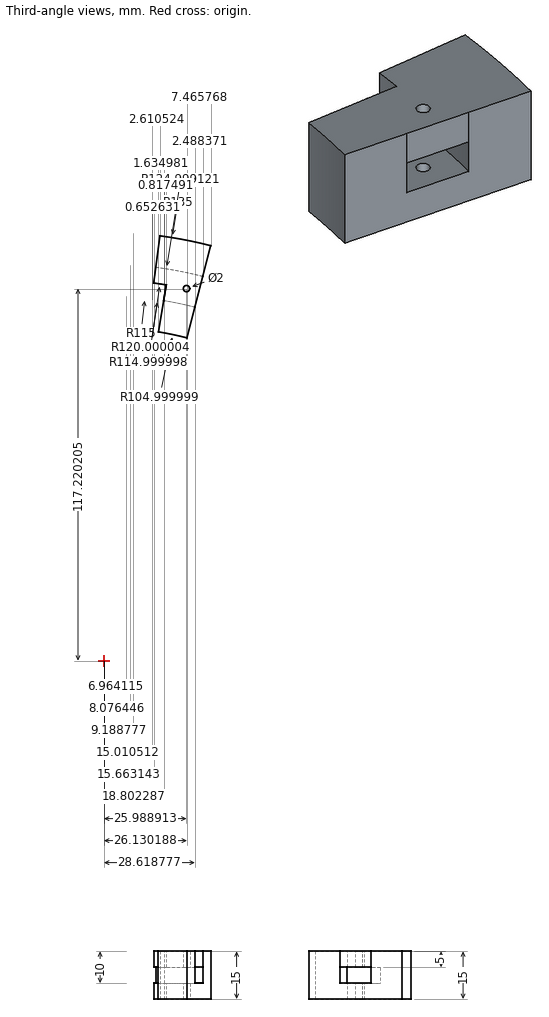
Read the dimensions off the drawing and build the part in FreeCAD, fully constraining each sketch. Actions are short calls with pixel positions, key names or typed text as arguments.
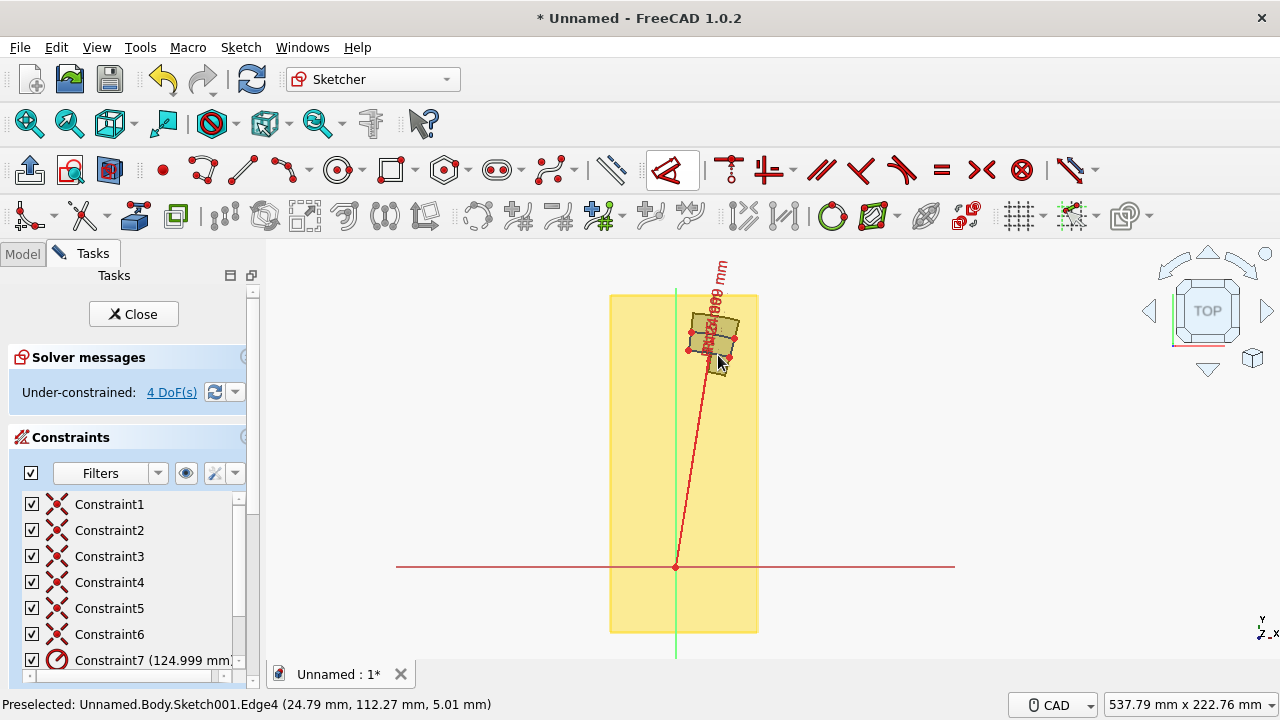
scroll(691, 332, up, 5)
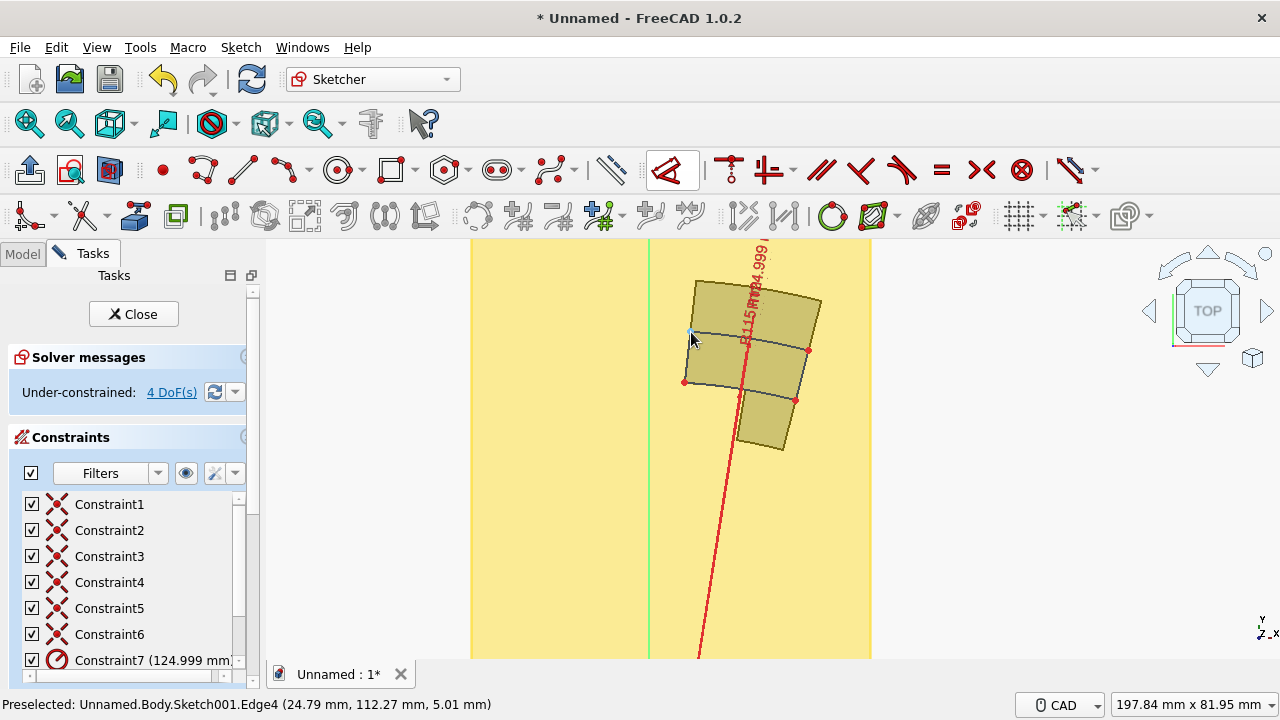
click(690, 332)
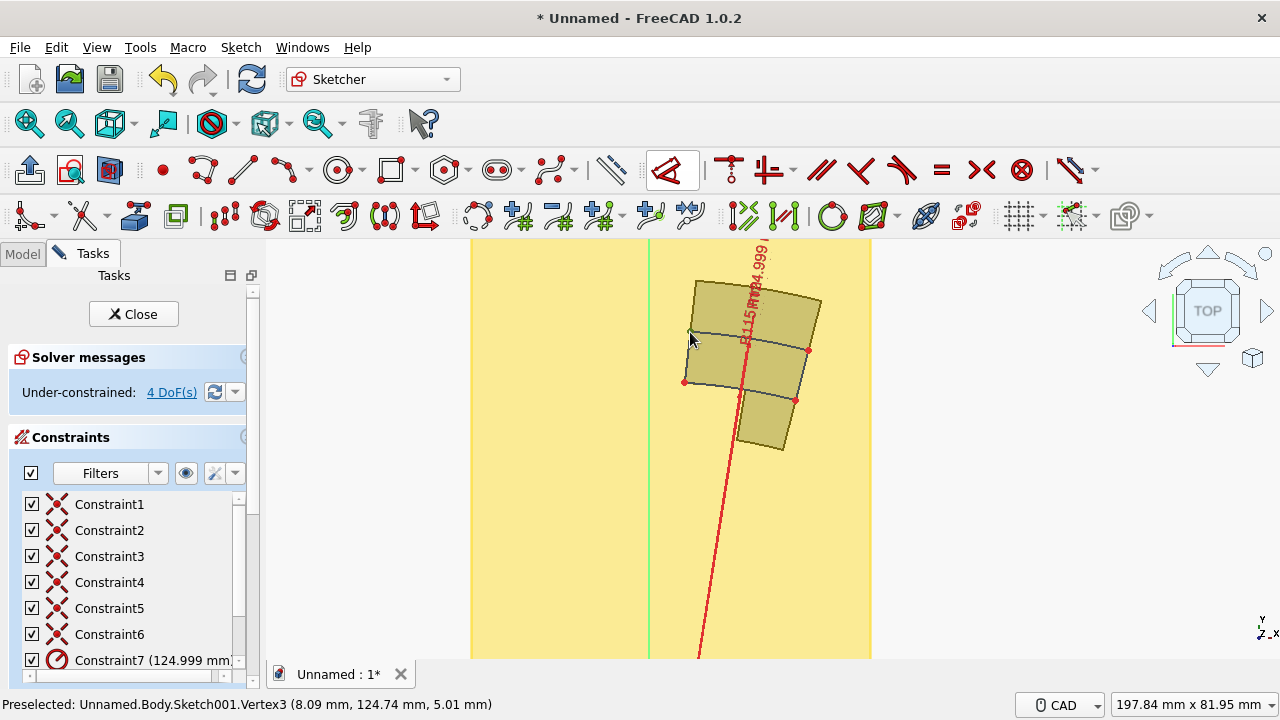
click(694, 170)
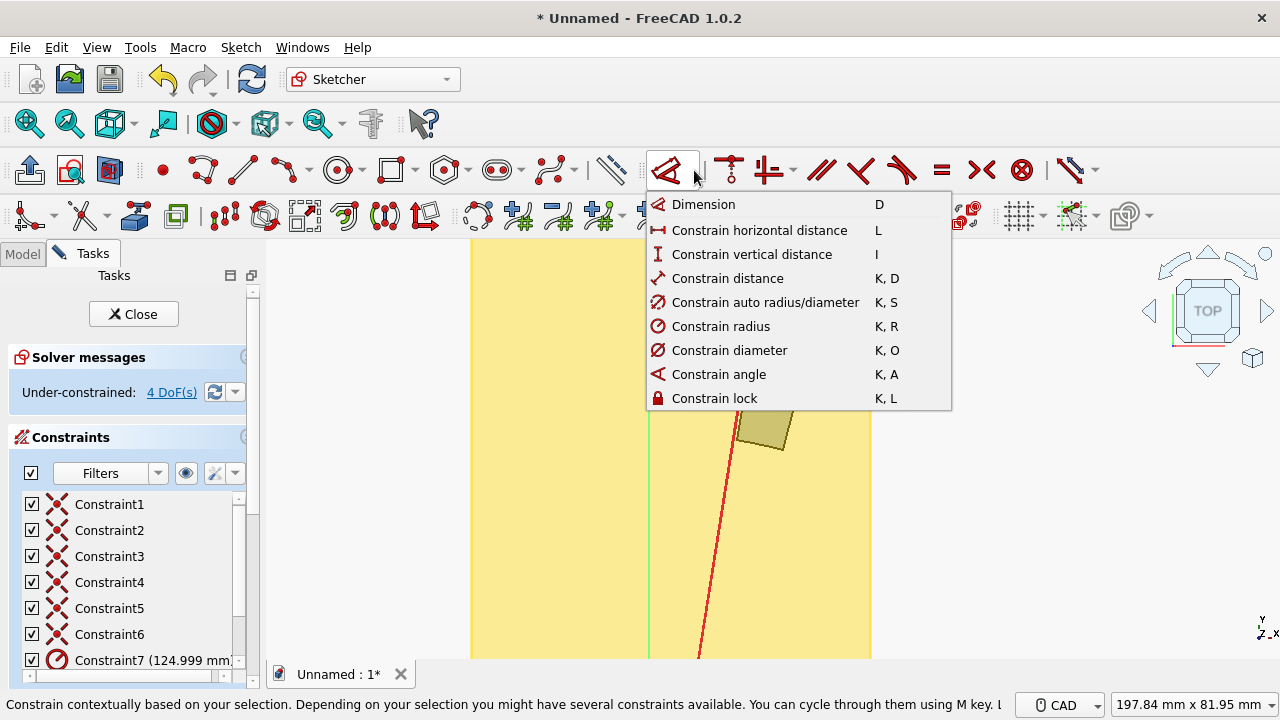
click(799, 230)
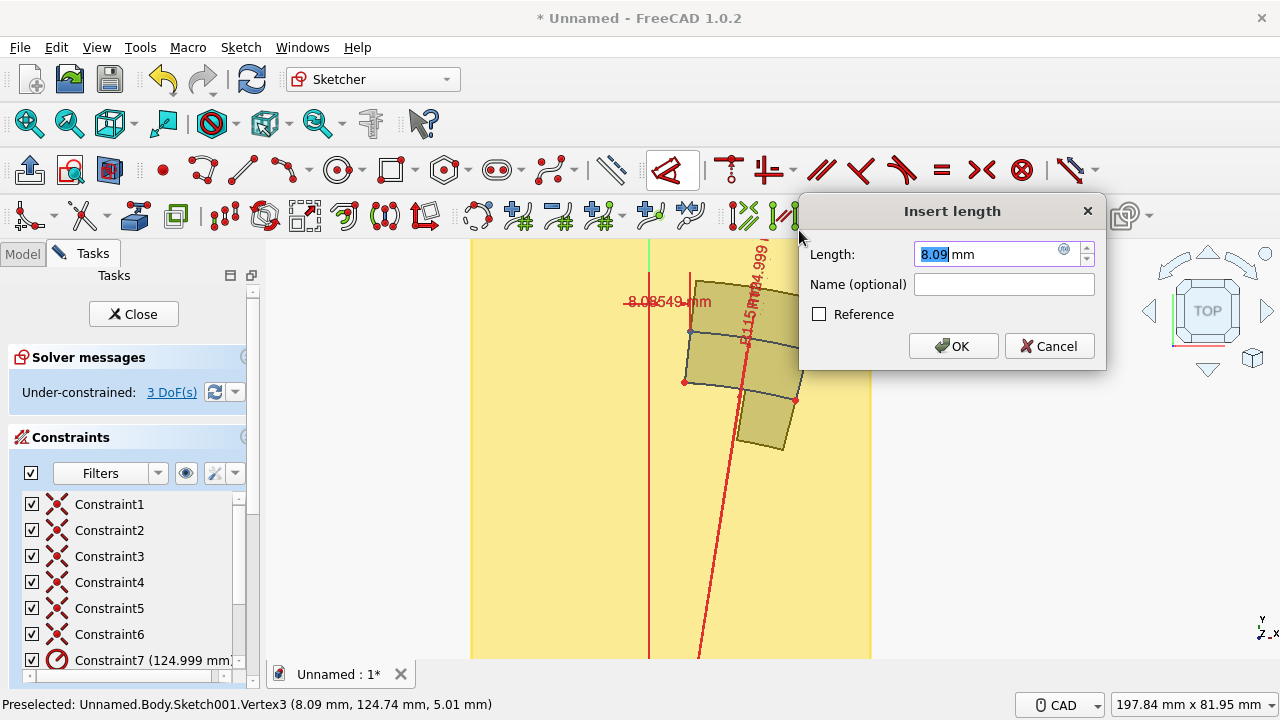
text(8.076446)
key(Return)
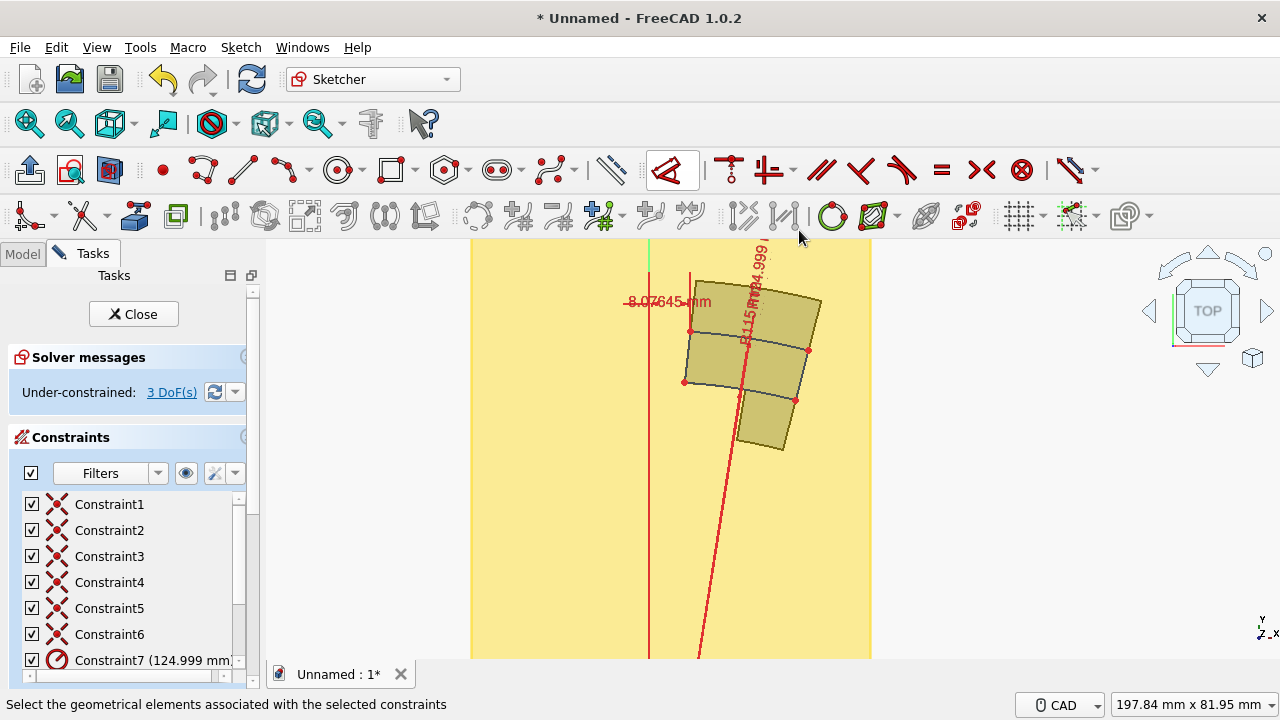
click(685, 383)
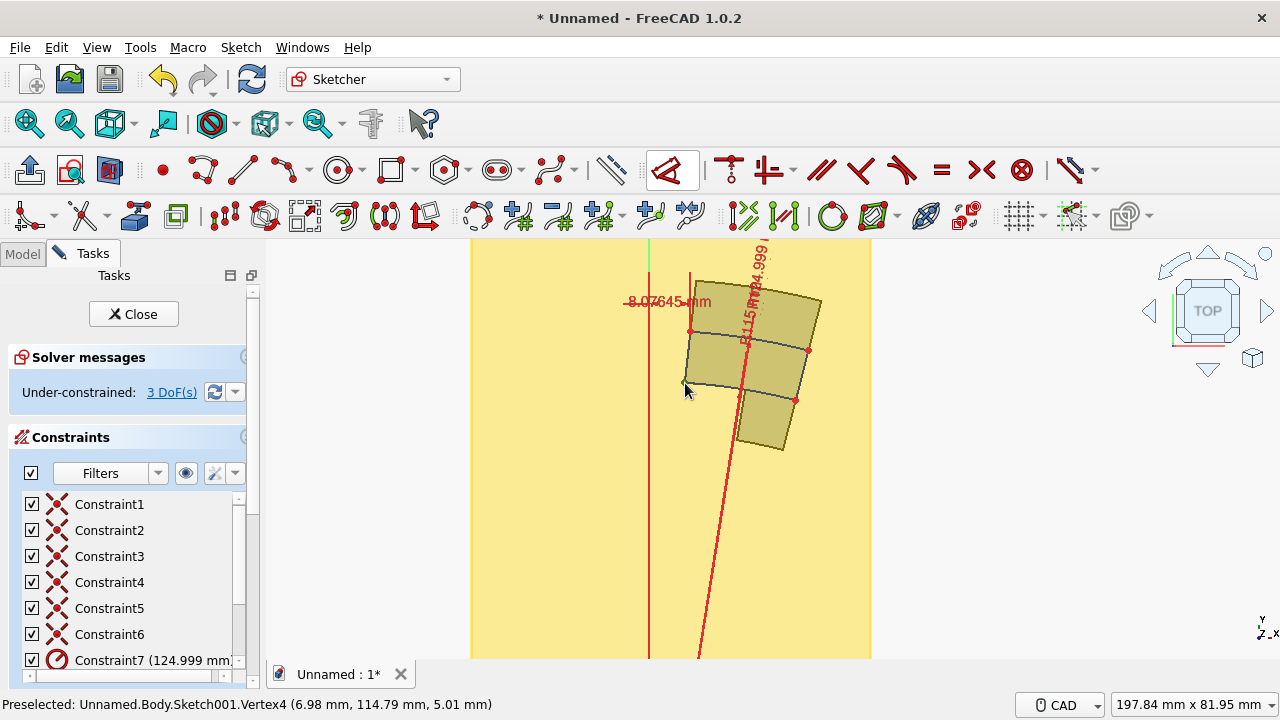
key(l)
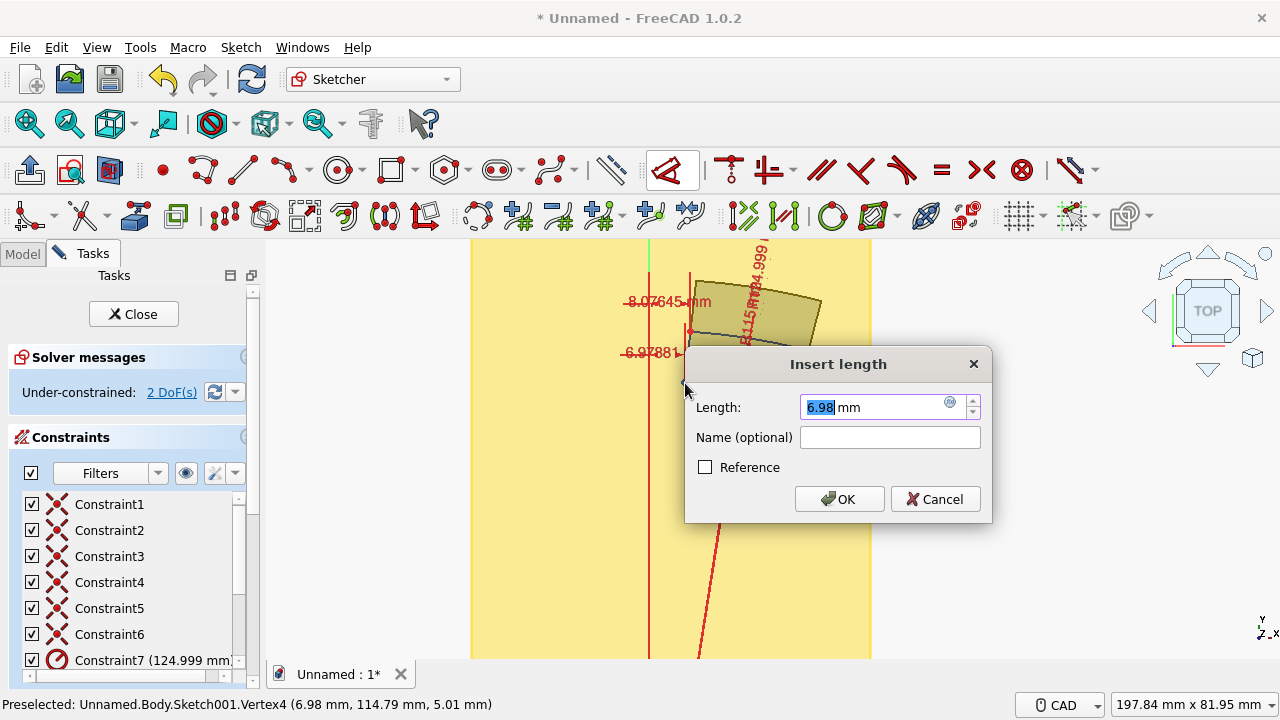
text(6.964115)
key(Return)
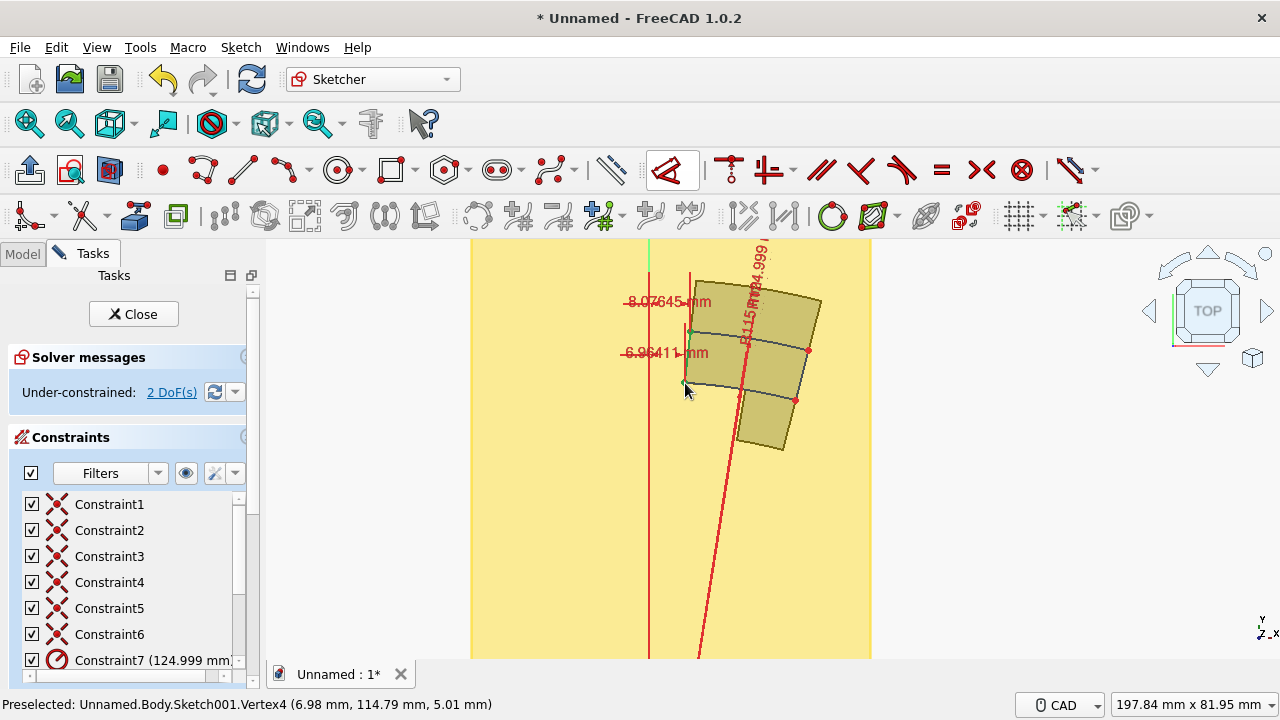
scroll(800, 385, up, 6)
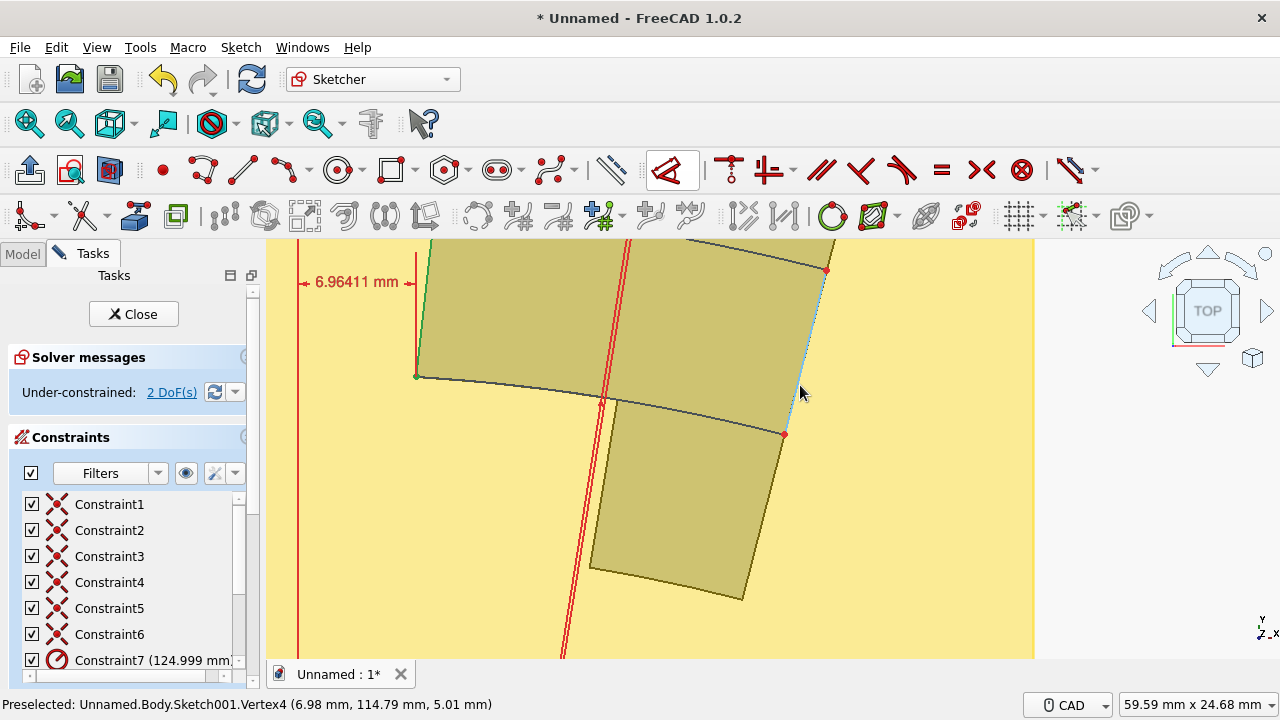
click(797, 385)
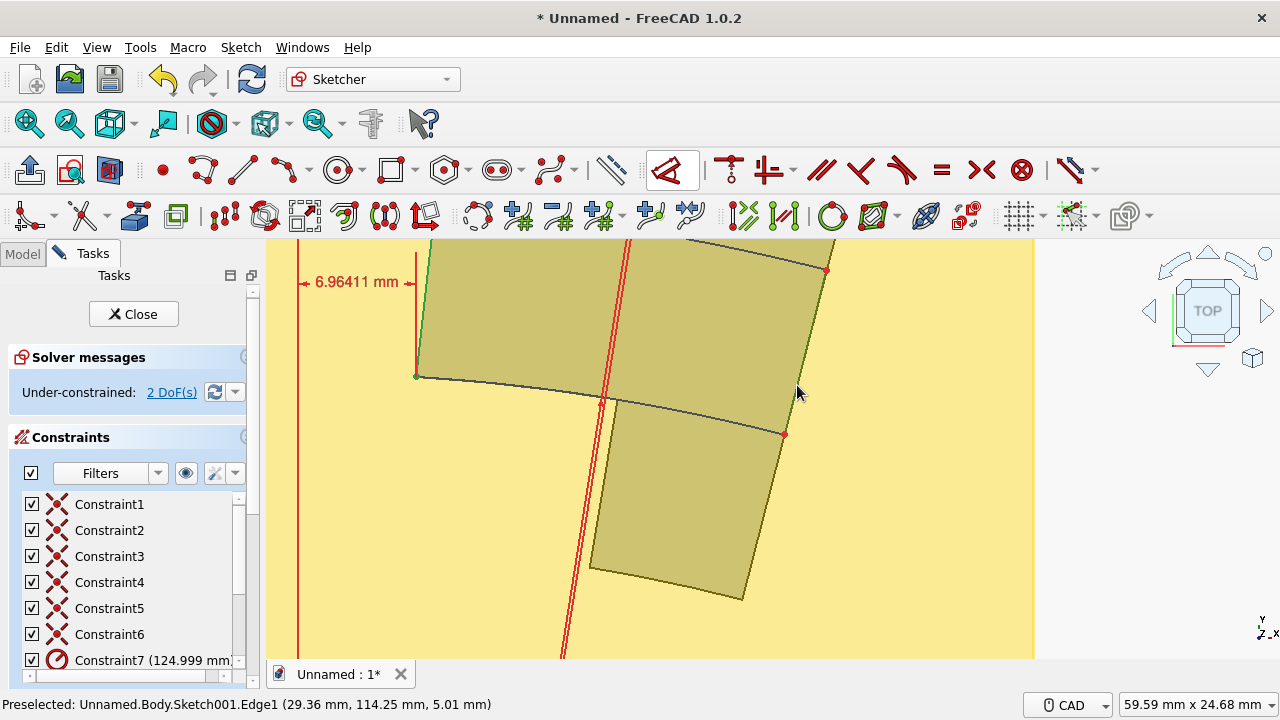
key(l)